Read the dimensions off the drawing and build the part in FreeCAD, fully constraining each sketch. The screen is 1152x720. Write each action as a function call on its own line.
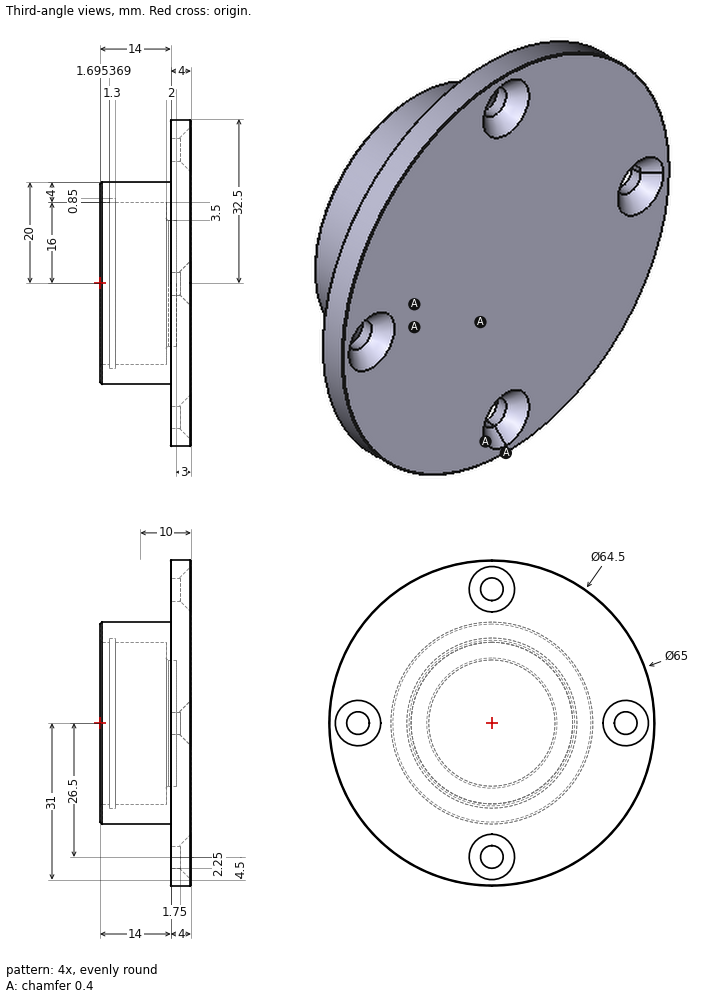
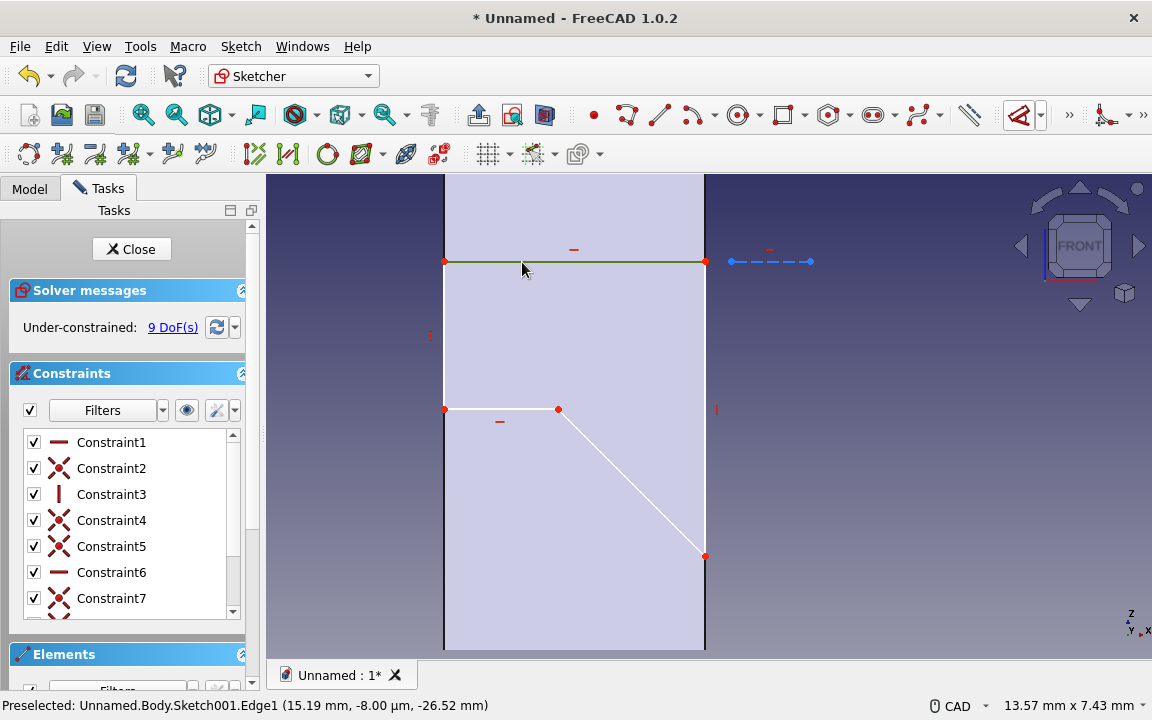
click(1040, 116)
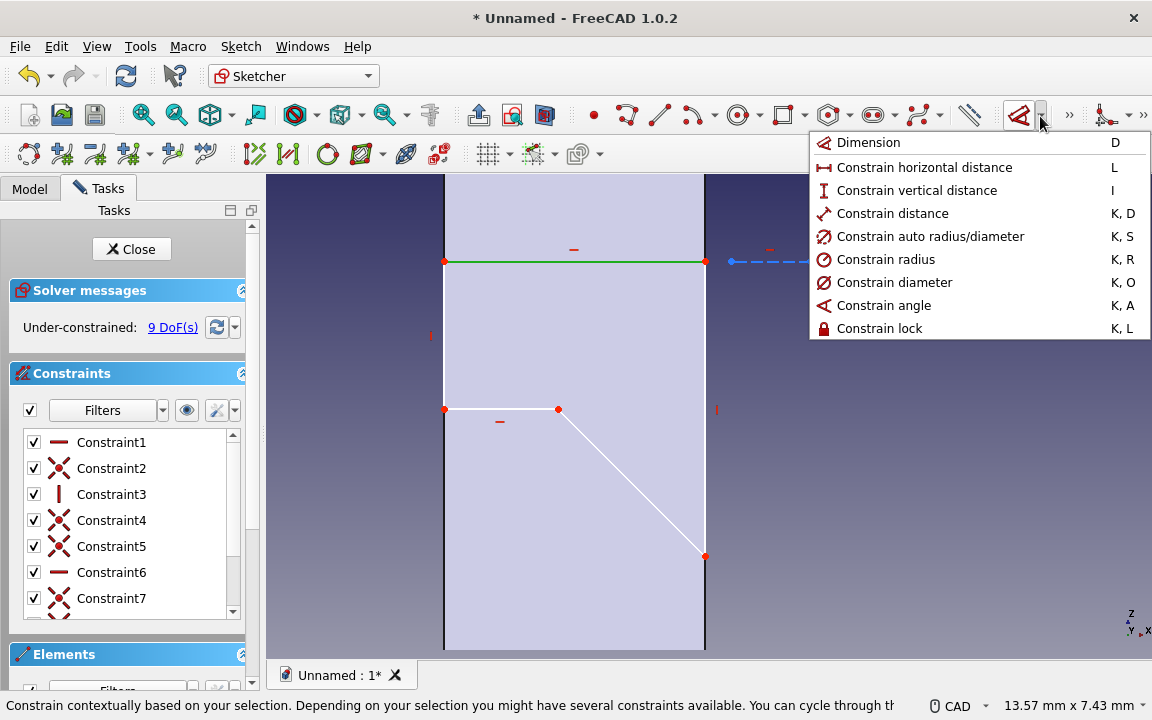
click(980, 168)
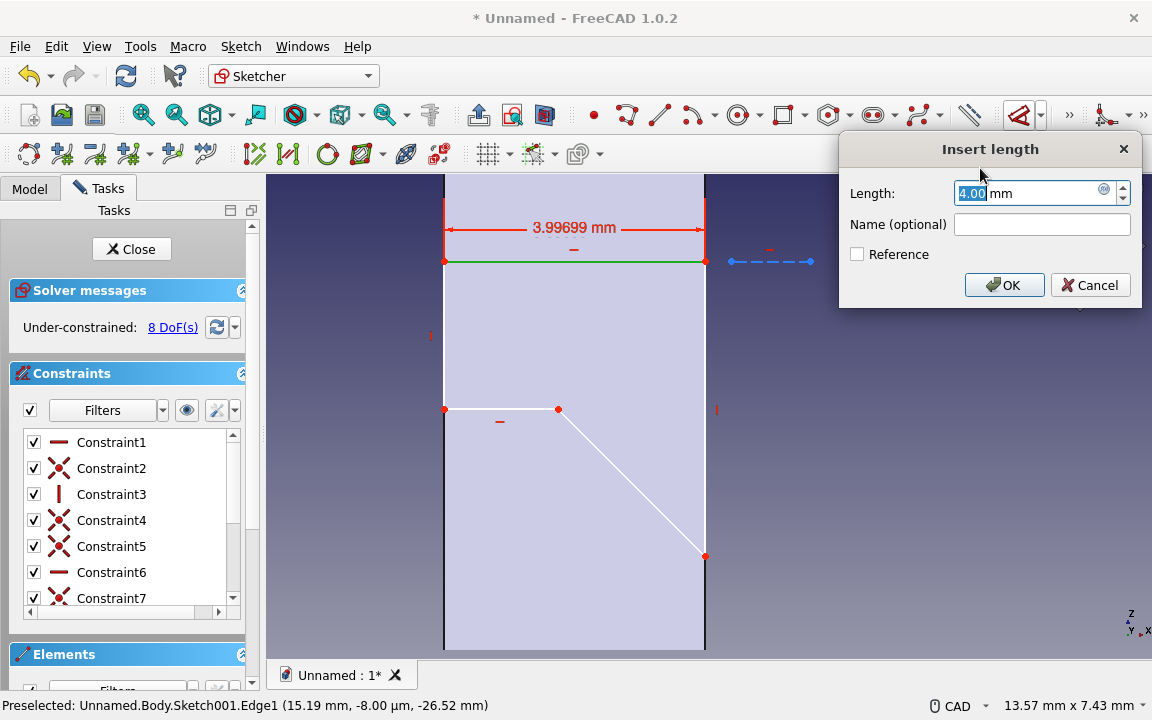
text(4)
key(Return)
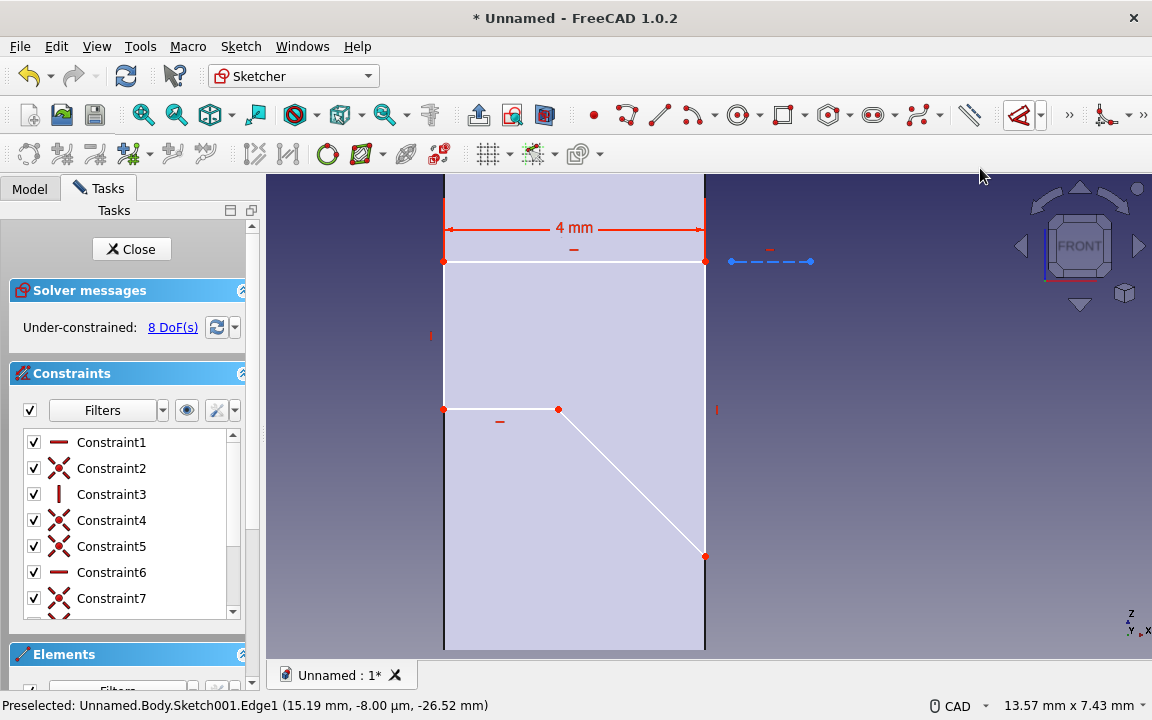
click(705, 350)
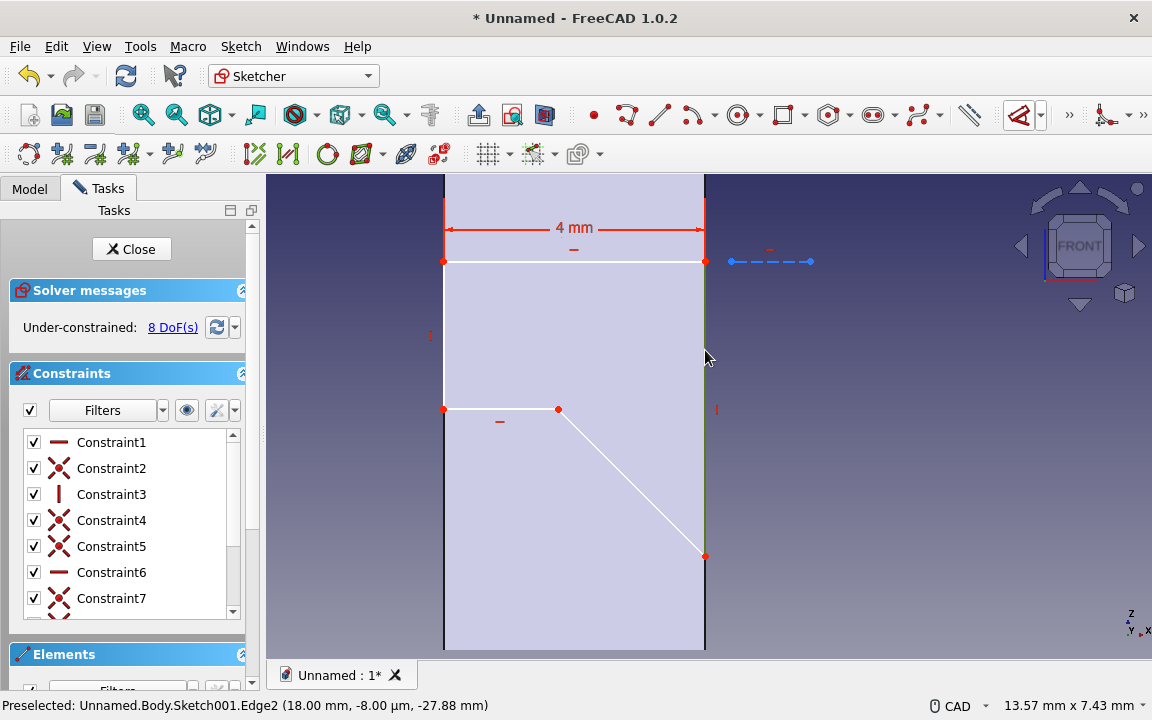
click(1040, 116)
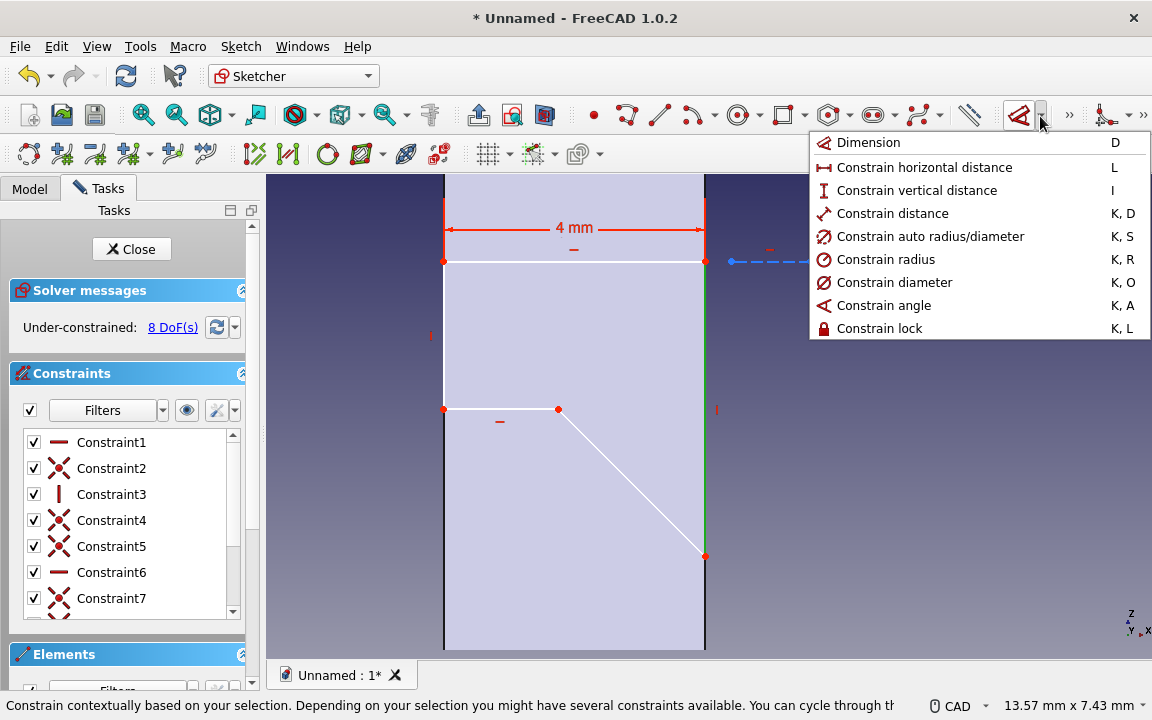
click(980, 190)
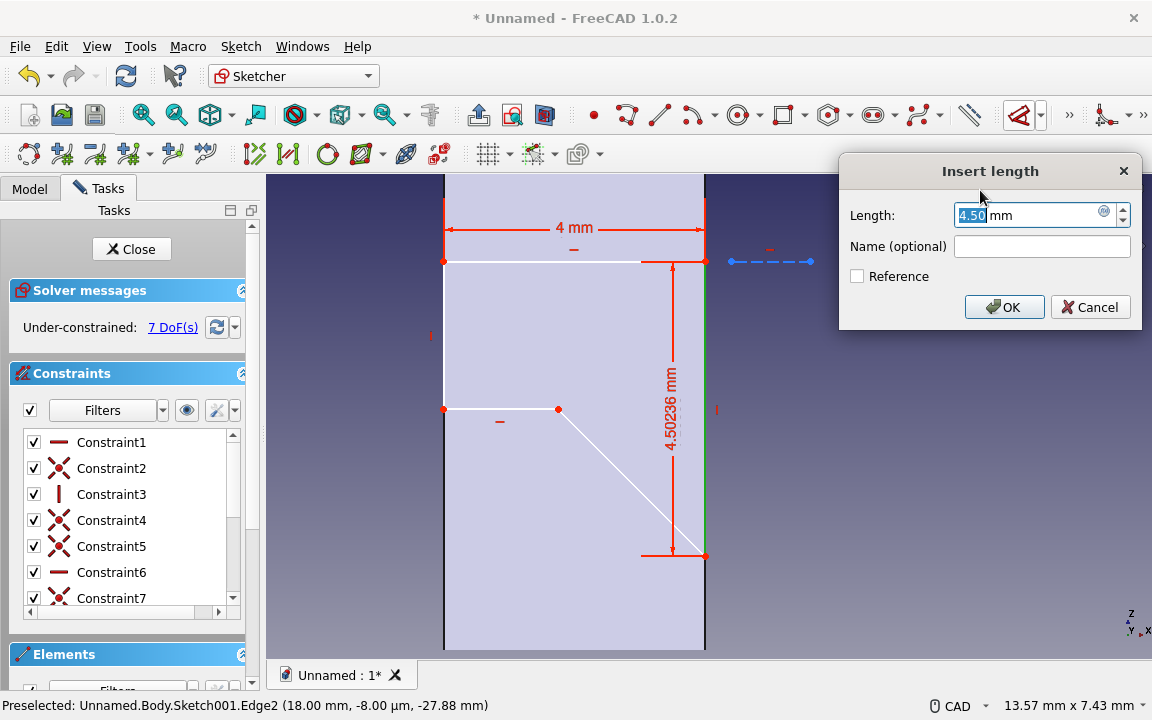
text(4.5)
key(Return)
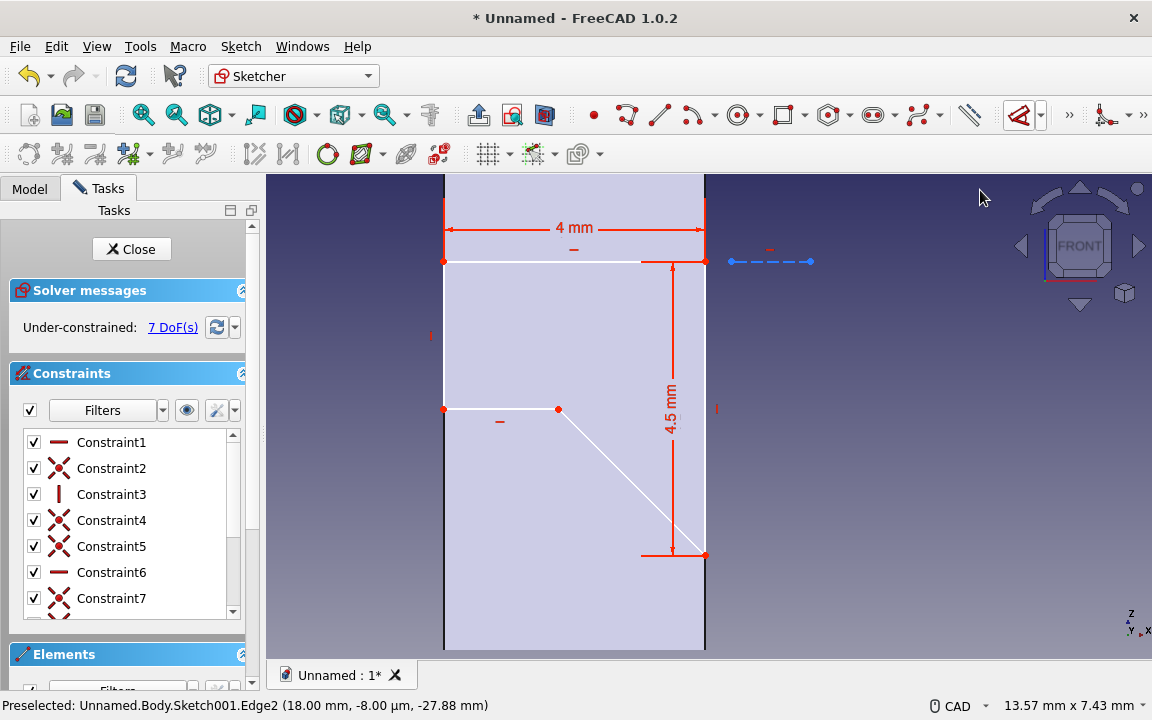
click(444, 262)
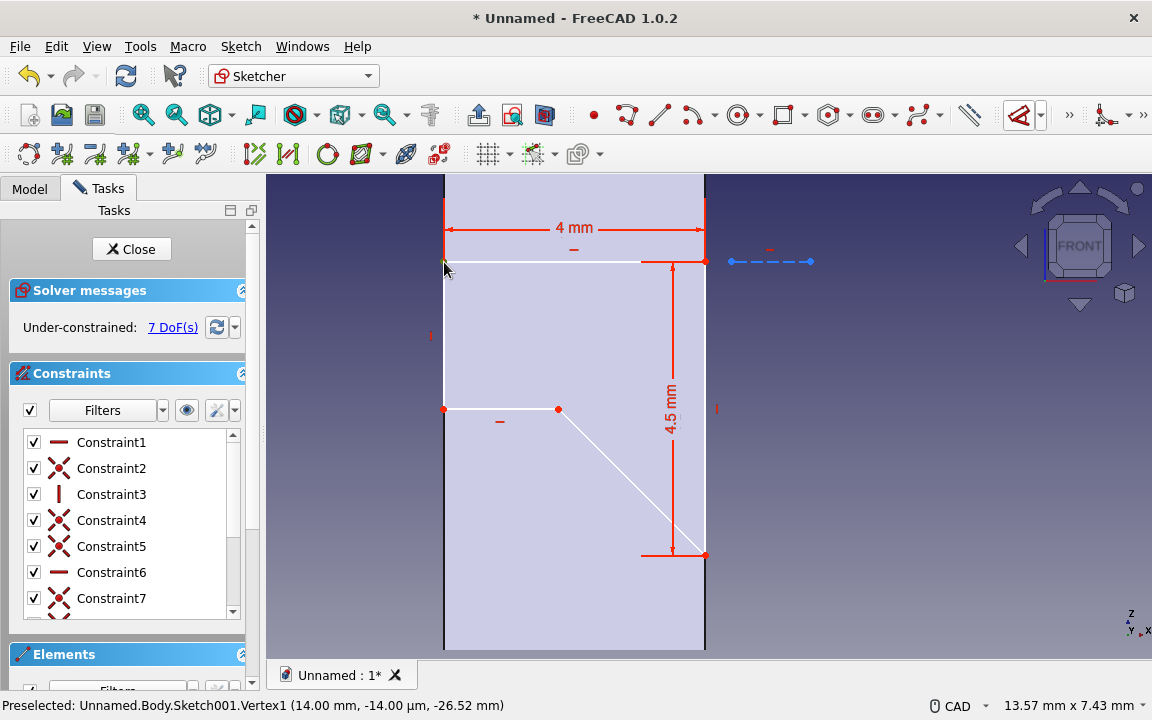
key(l)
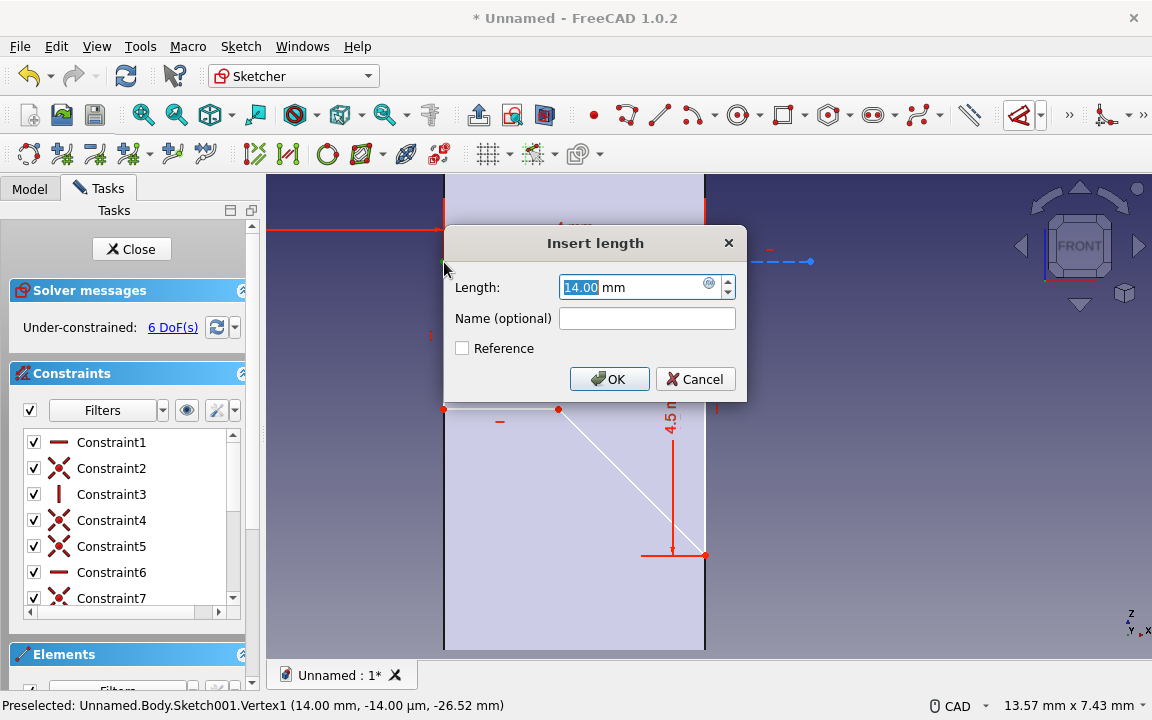
text(14)
key(Return)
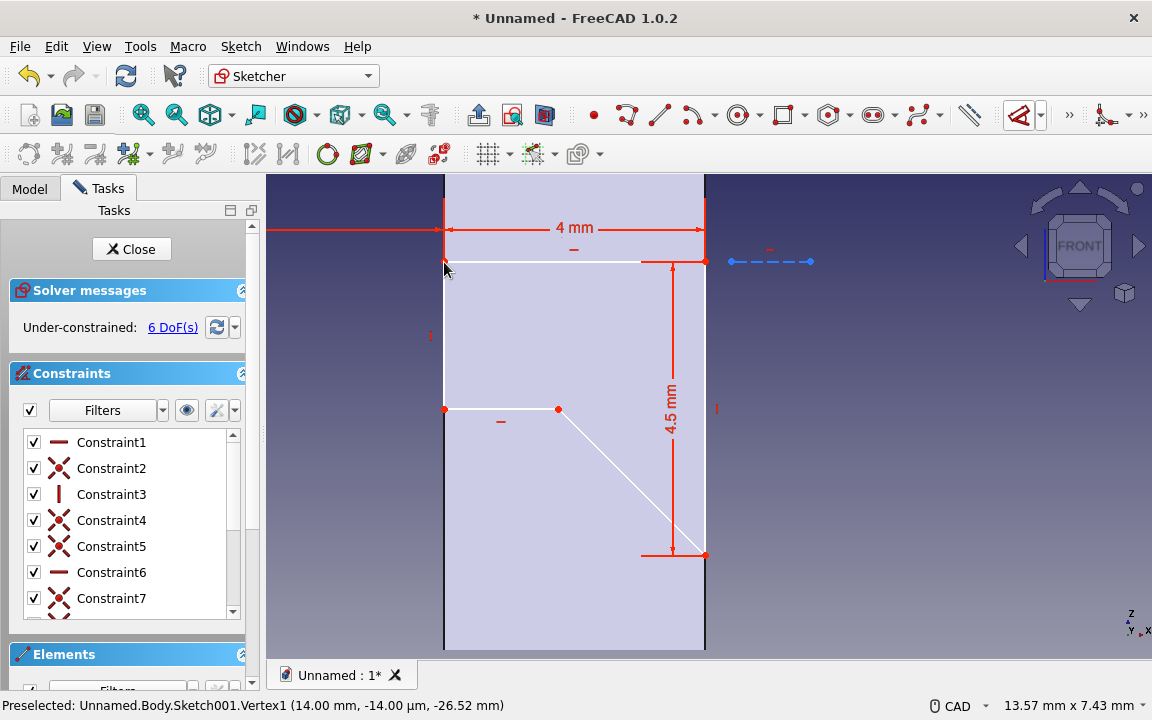
click(705, 556)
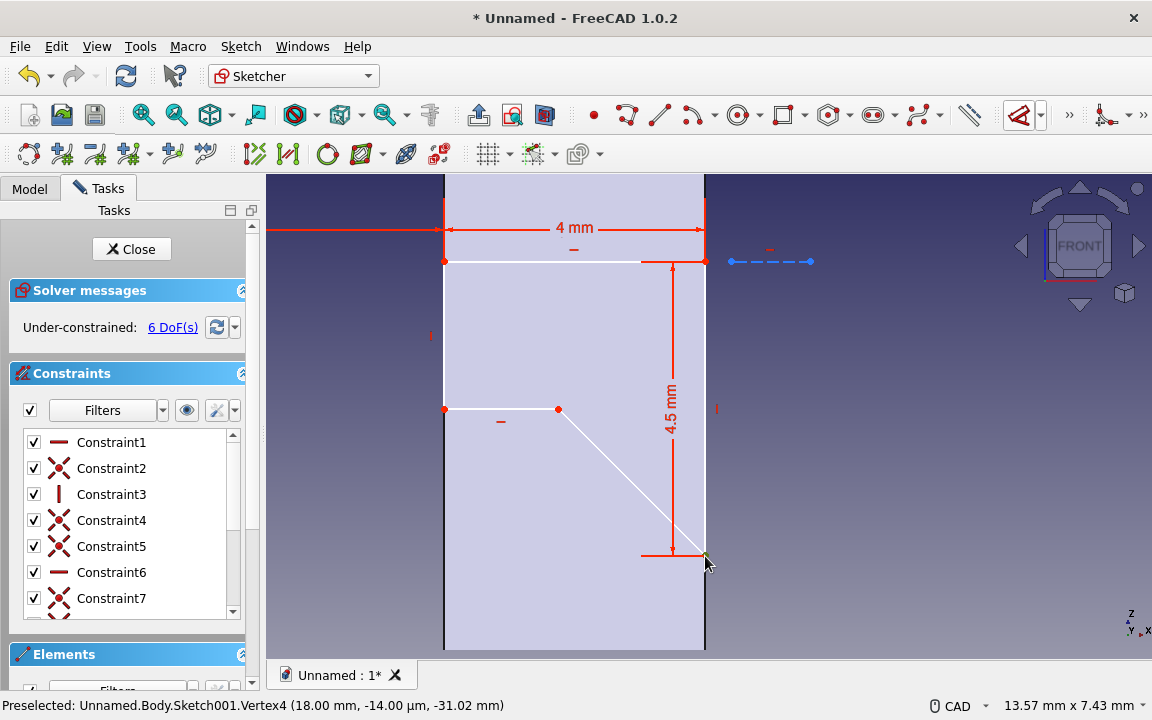
click(1040, 116)